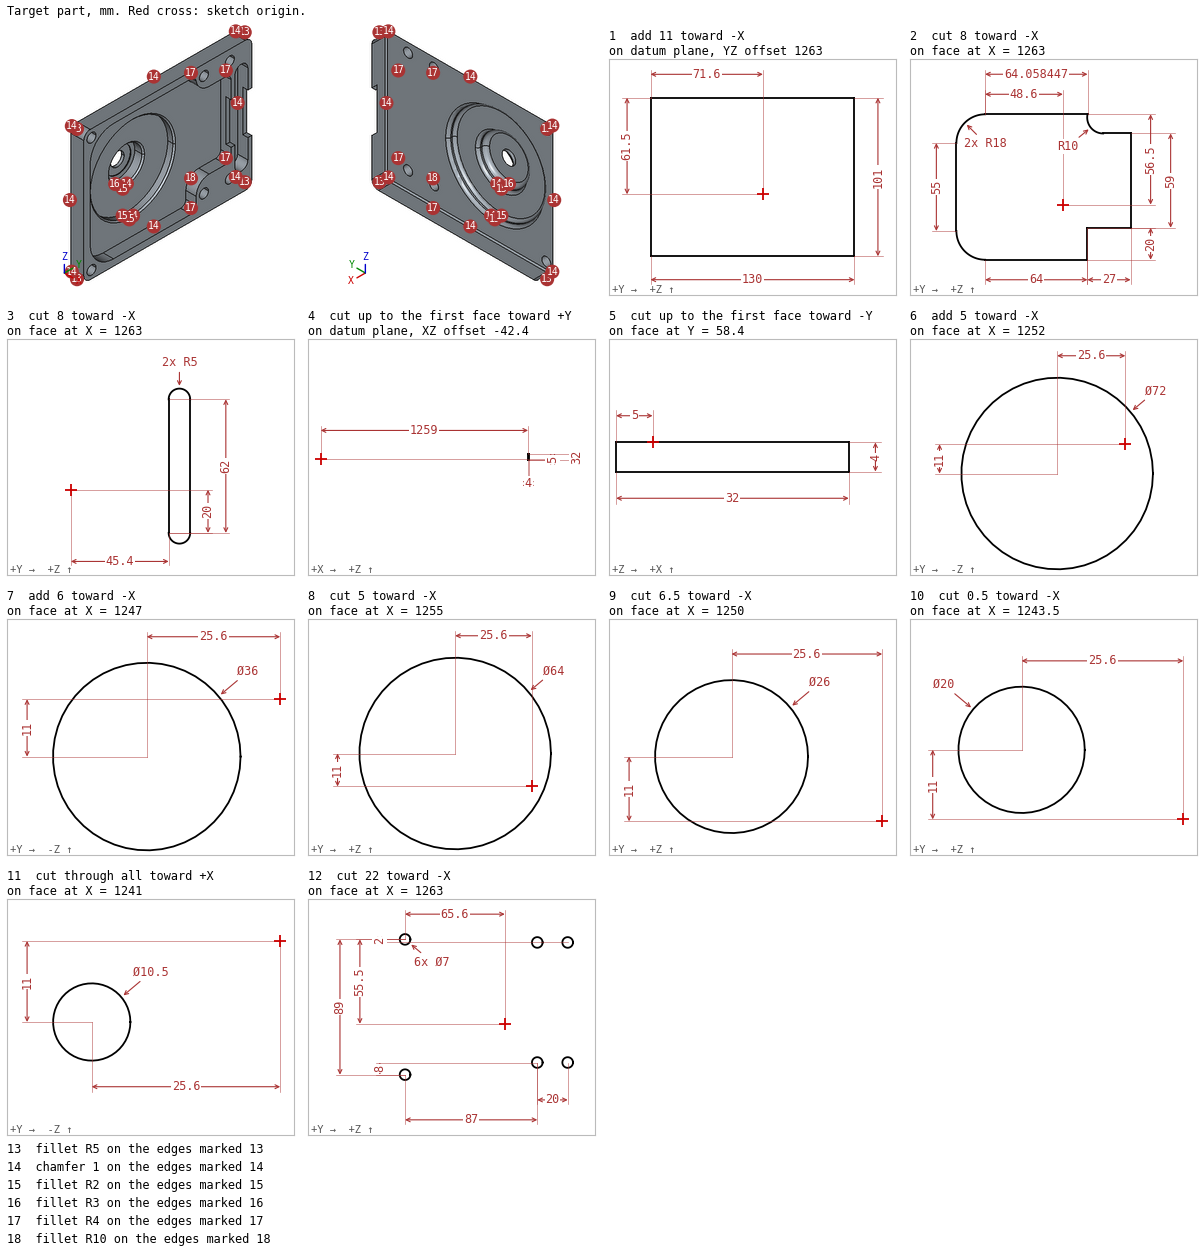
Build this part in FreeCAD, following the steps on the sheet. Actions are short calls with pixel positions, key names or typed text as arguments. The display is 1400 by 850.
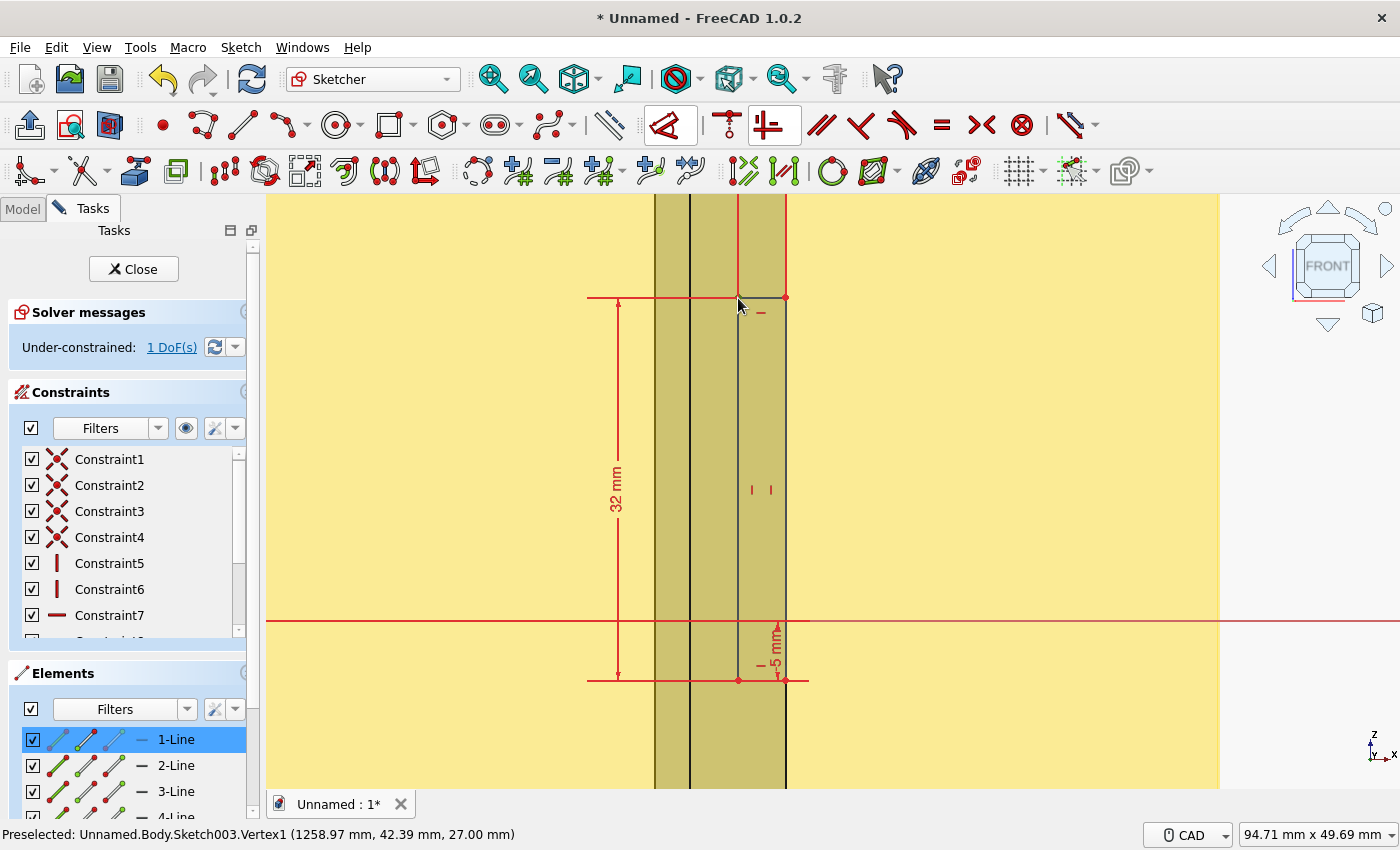
key(l)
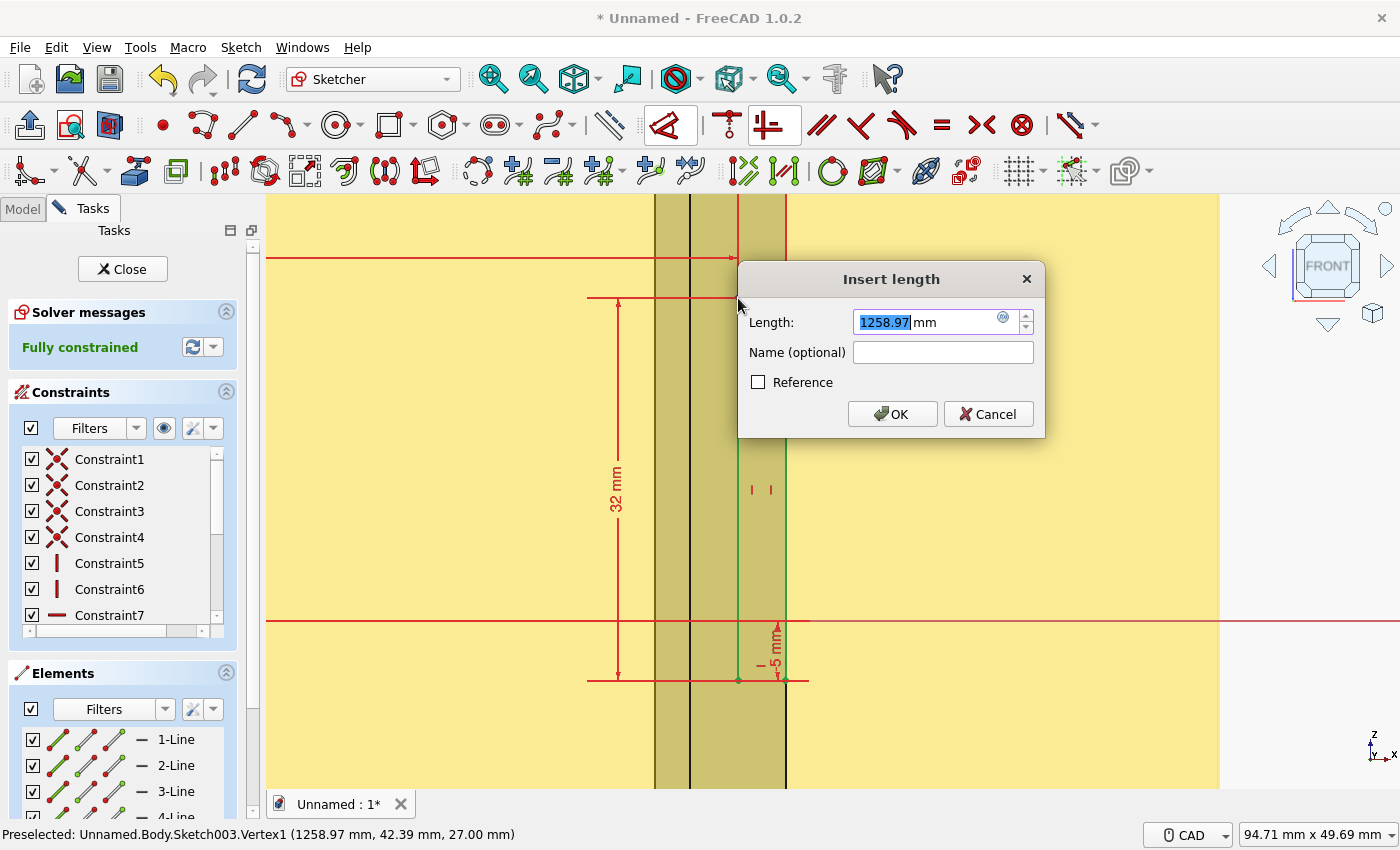
text(1259)
key(Return)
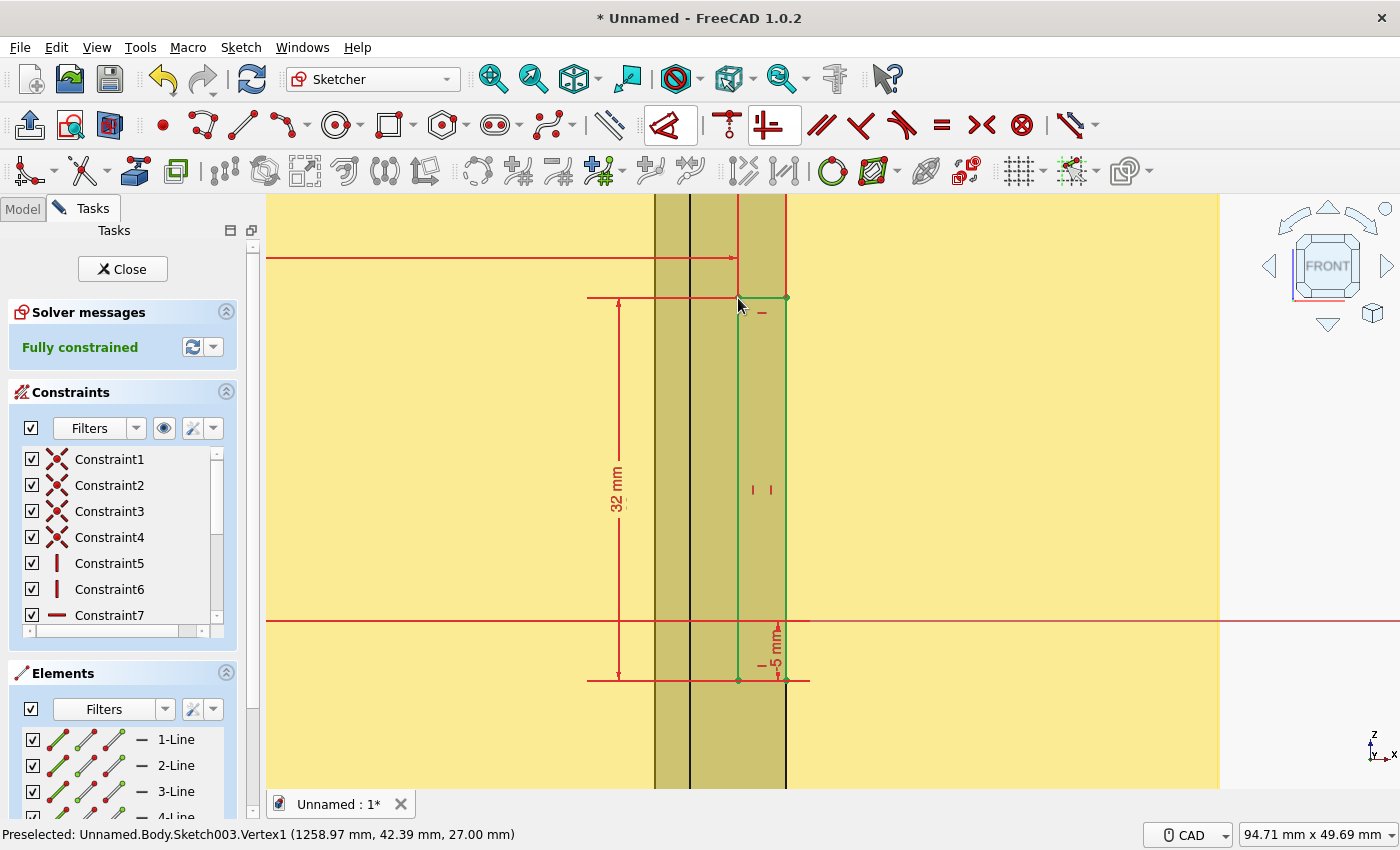
click(123, 269)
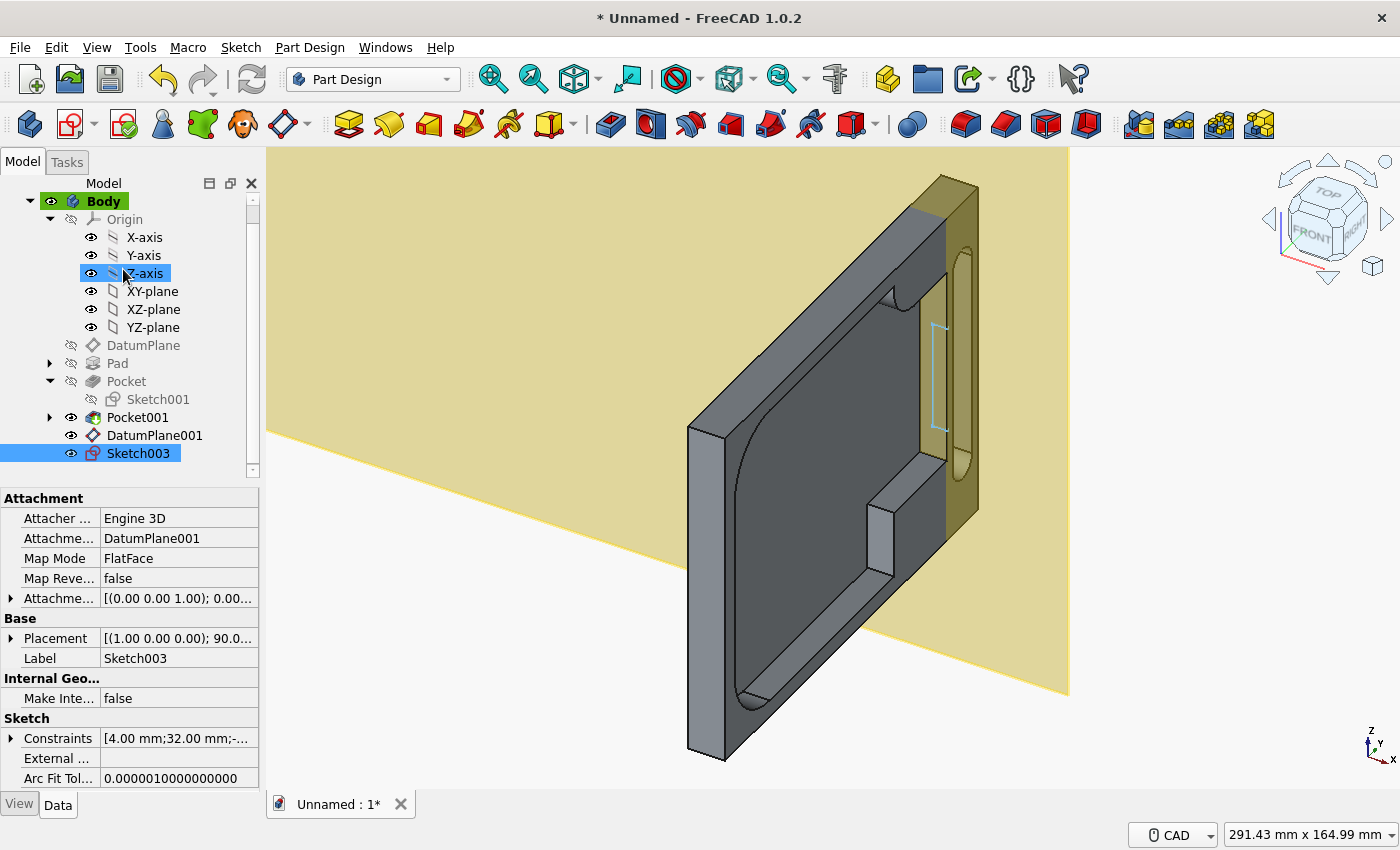
click(612, 124)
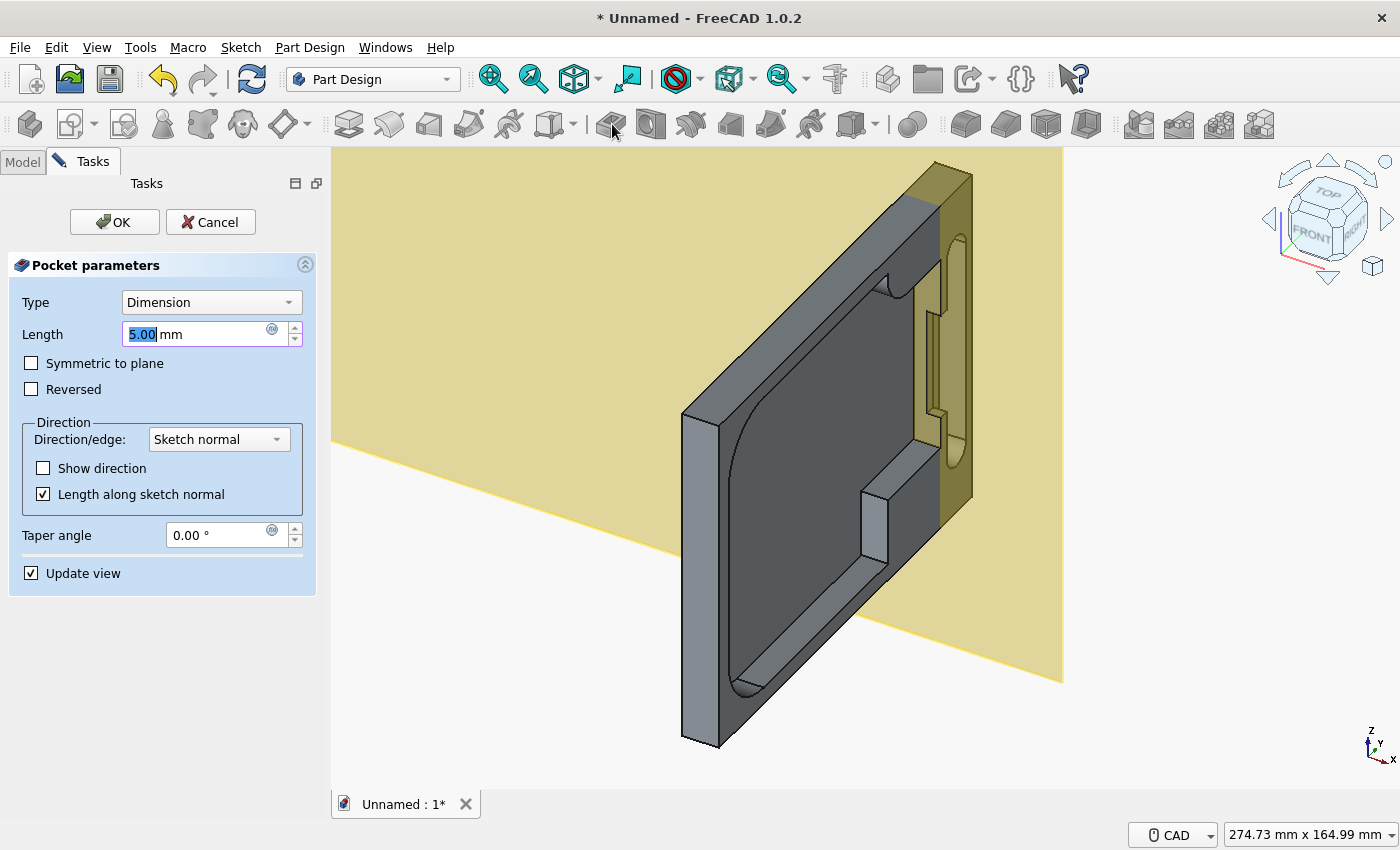
click(212, 302)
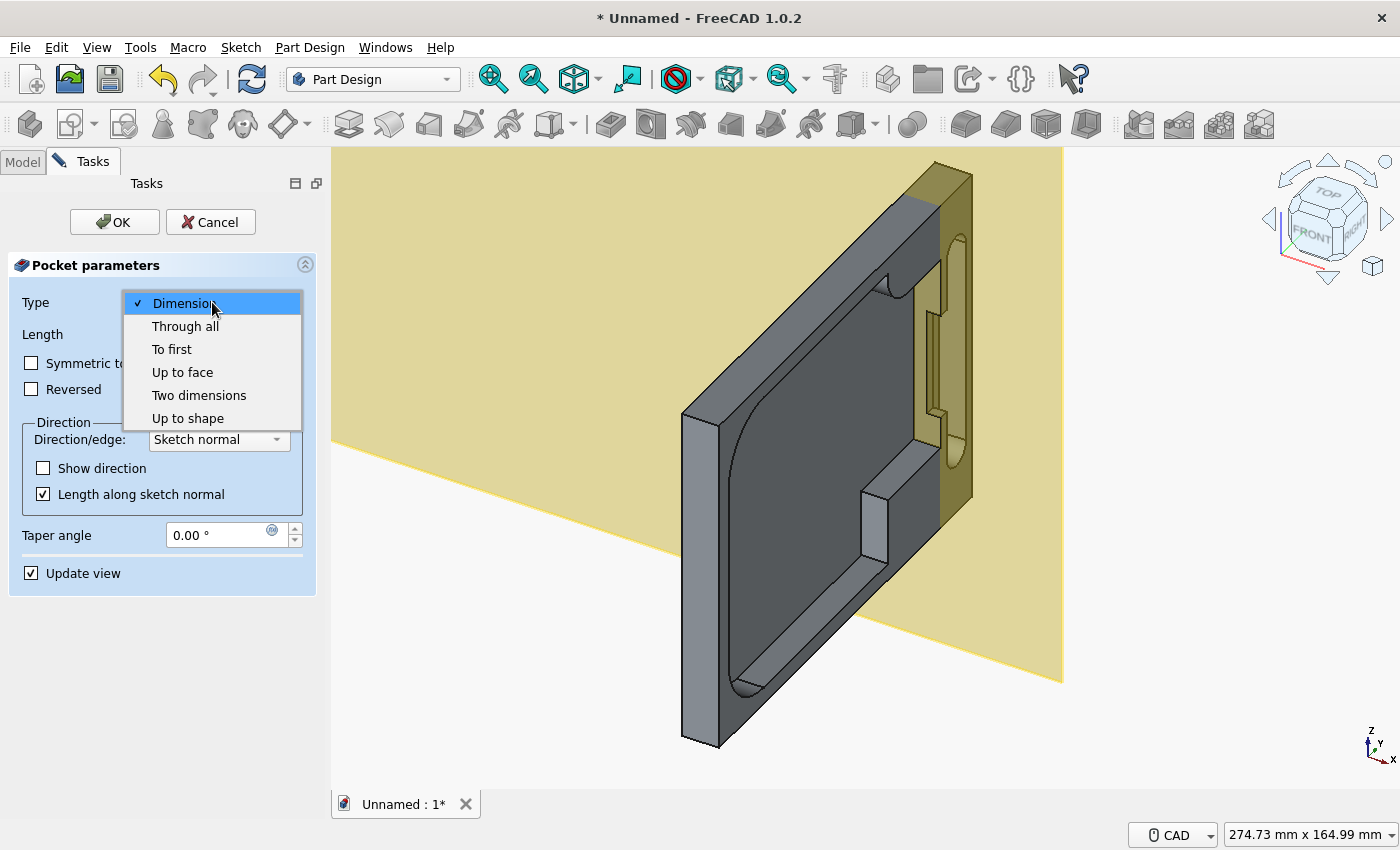
click(212, 350)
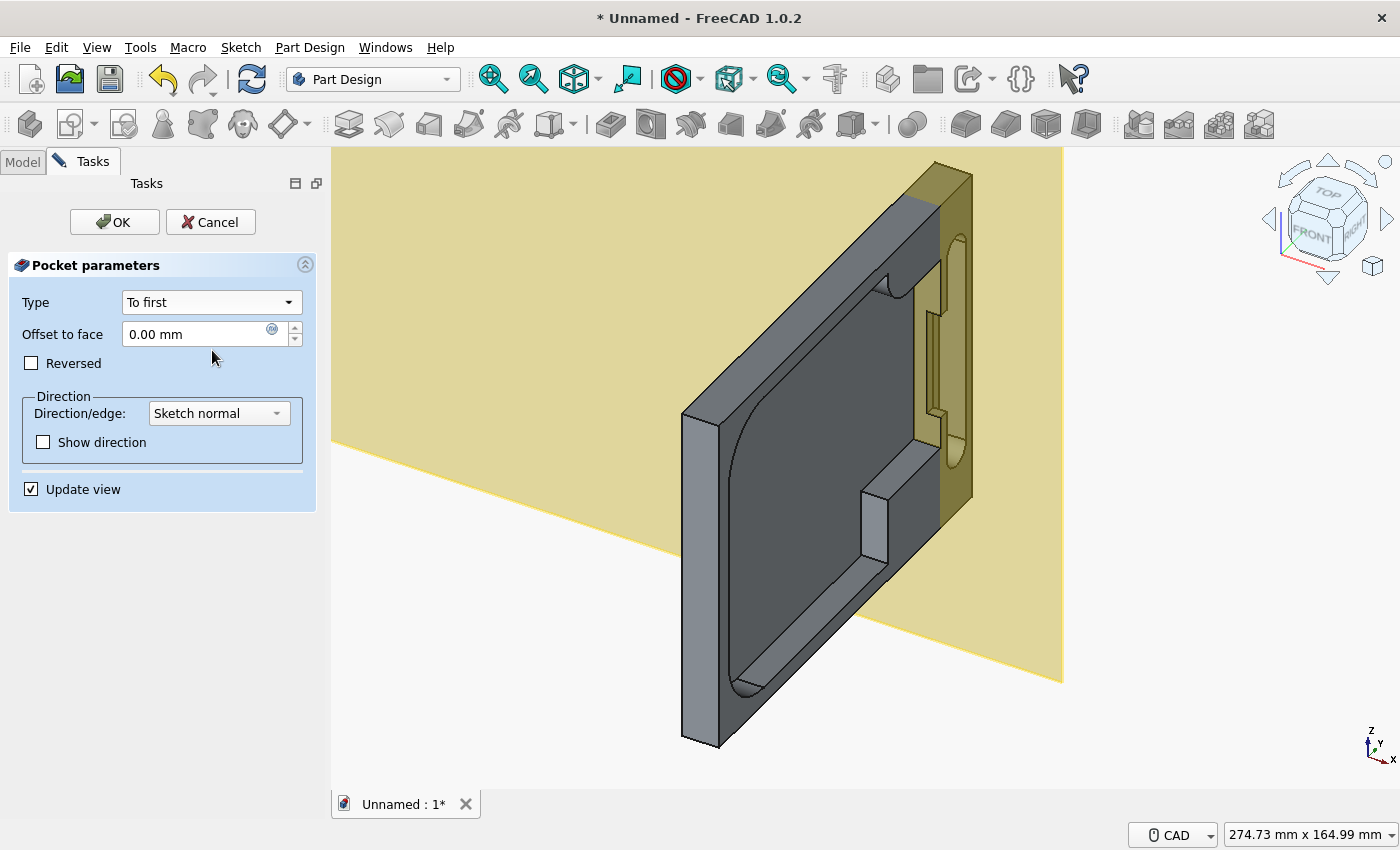
click(115, 222)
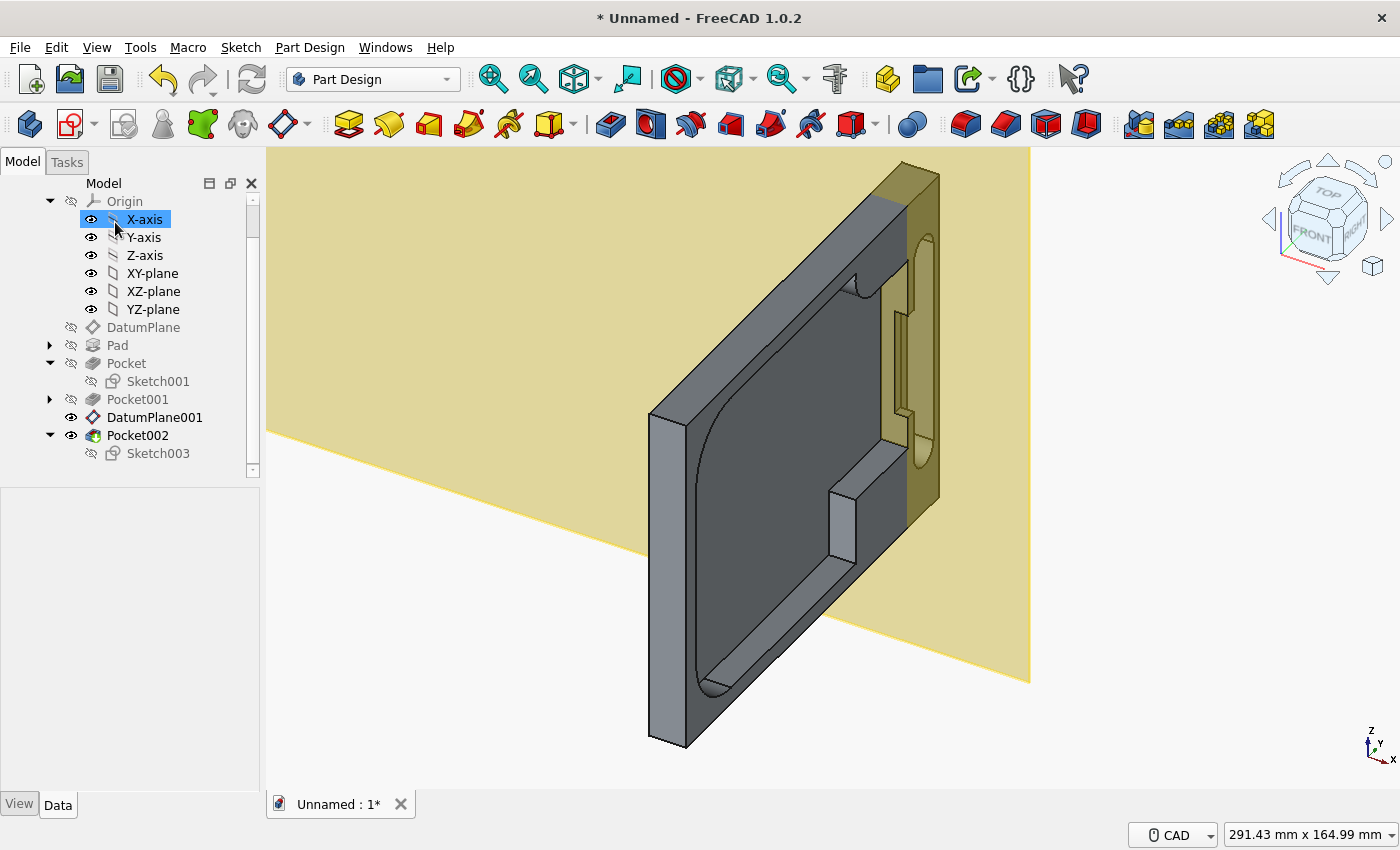
click(116, 417)
key(space)